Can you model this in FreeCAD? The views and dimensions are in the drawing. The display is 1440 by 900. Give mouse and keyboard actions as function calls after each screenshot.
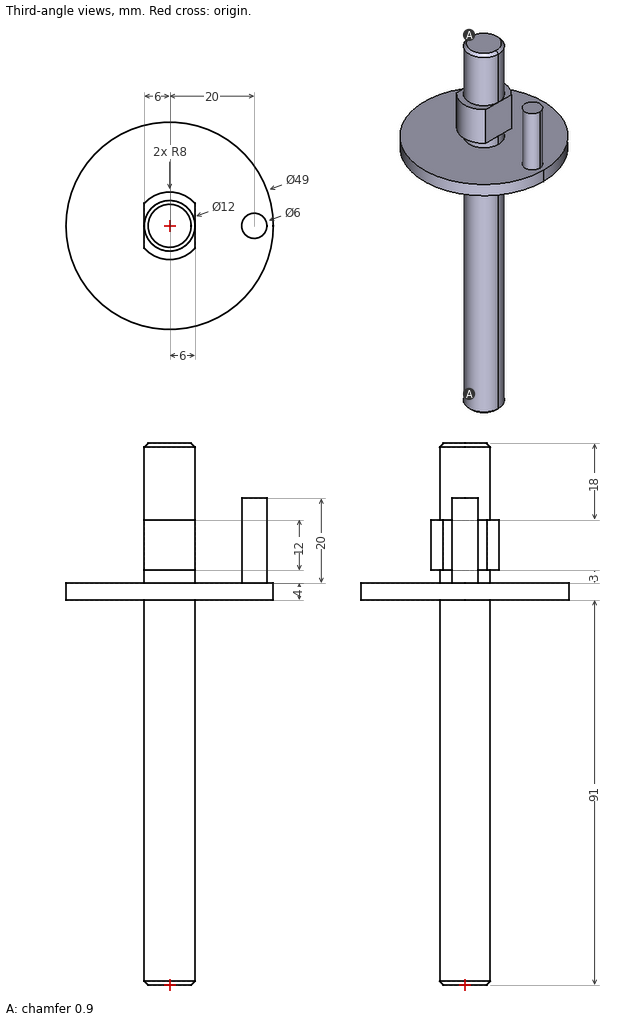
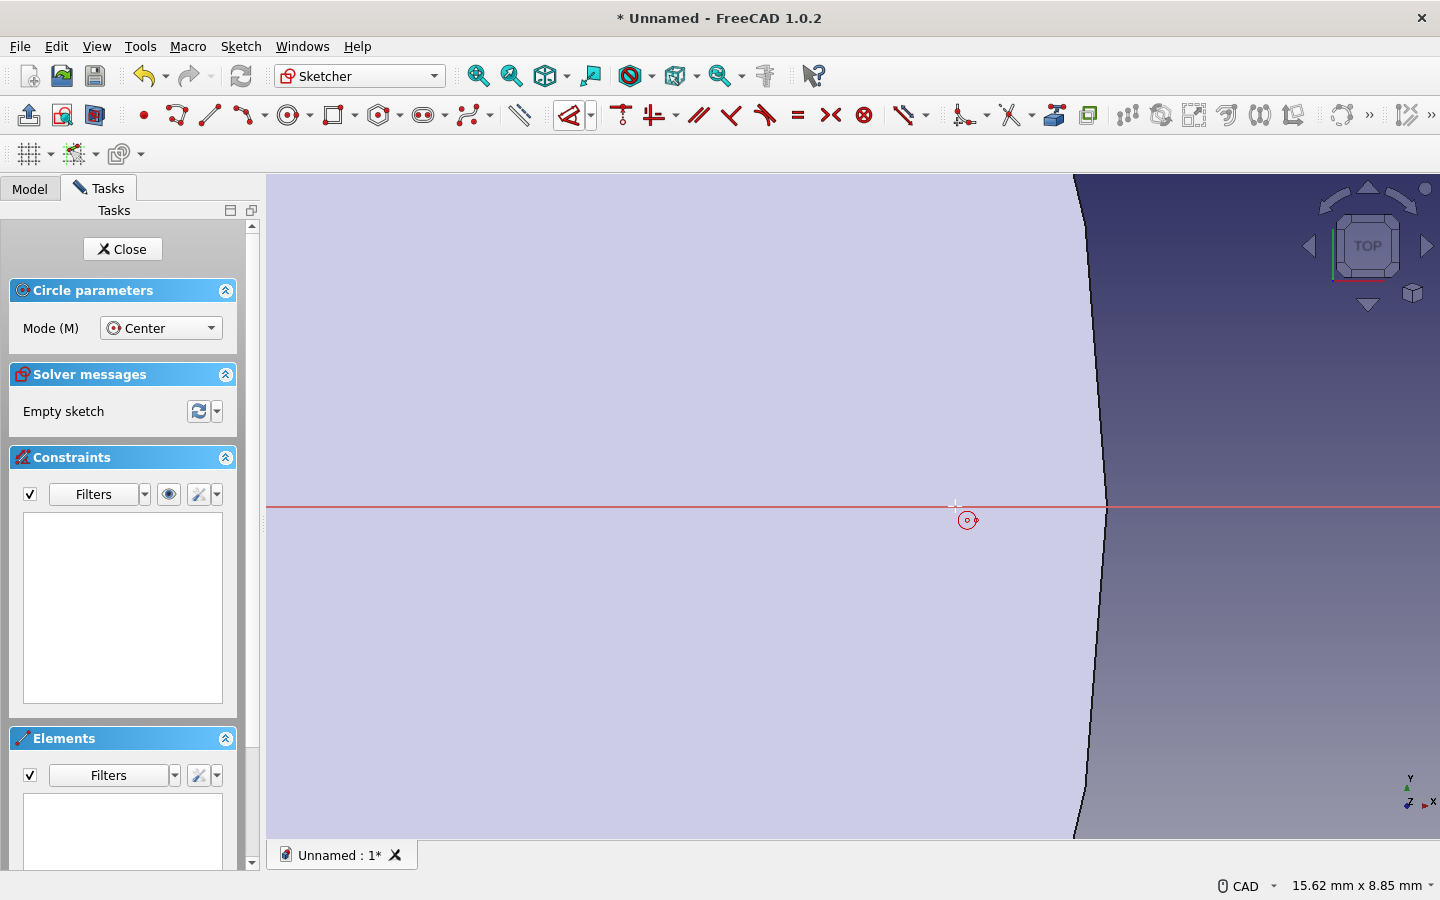
click(769, 506)
click(928, 347)
key(Escape)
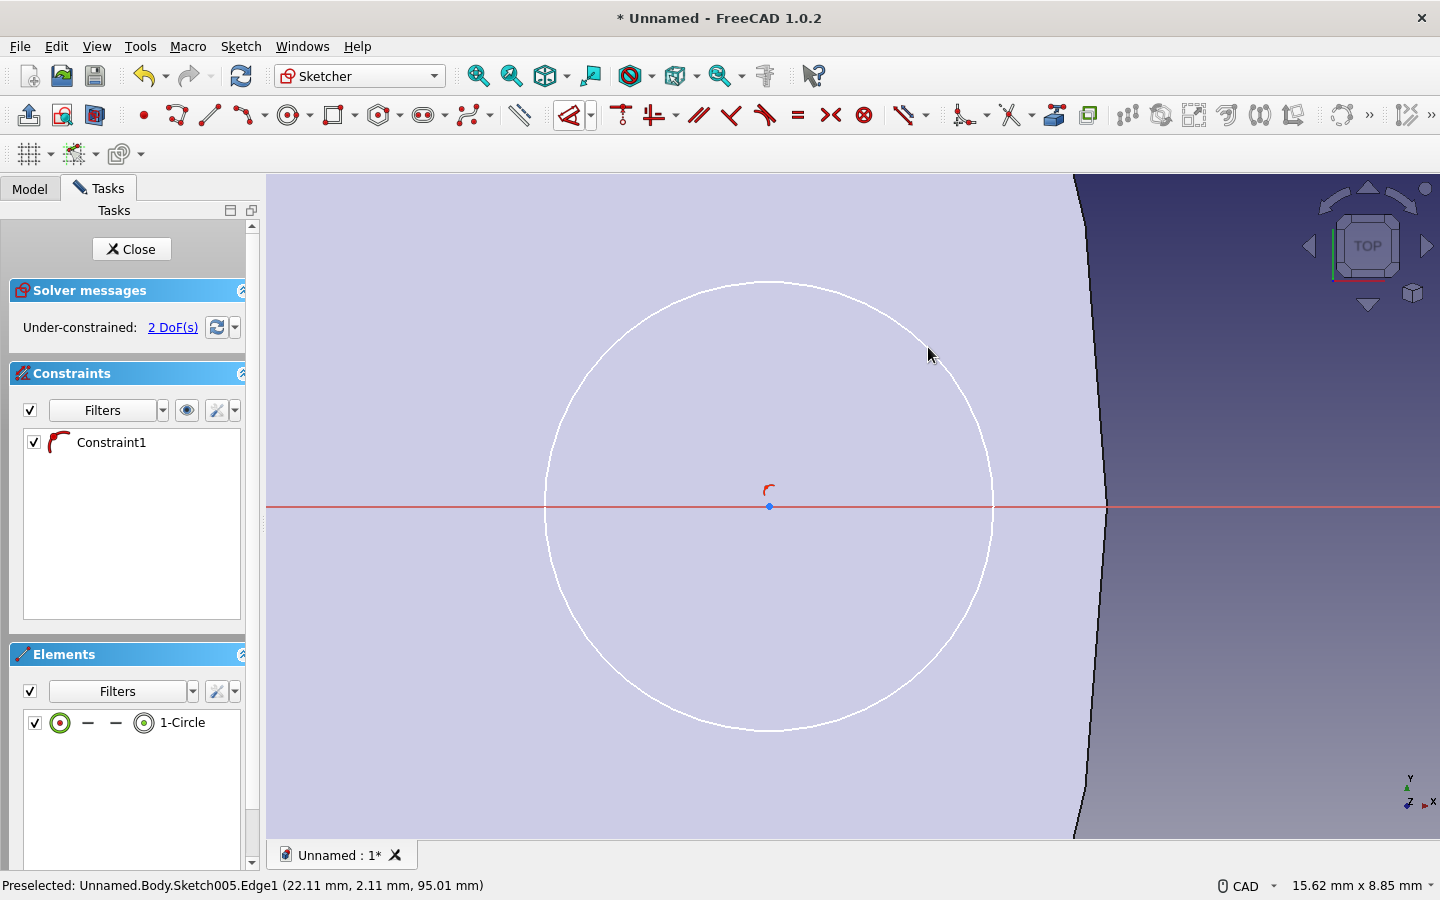
click(927, 347)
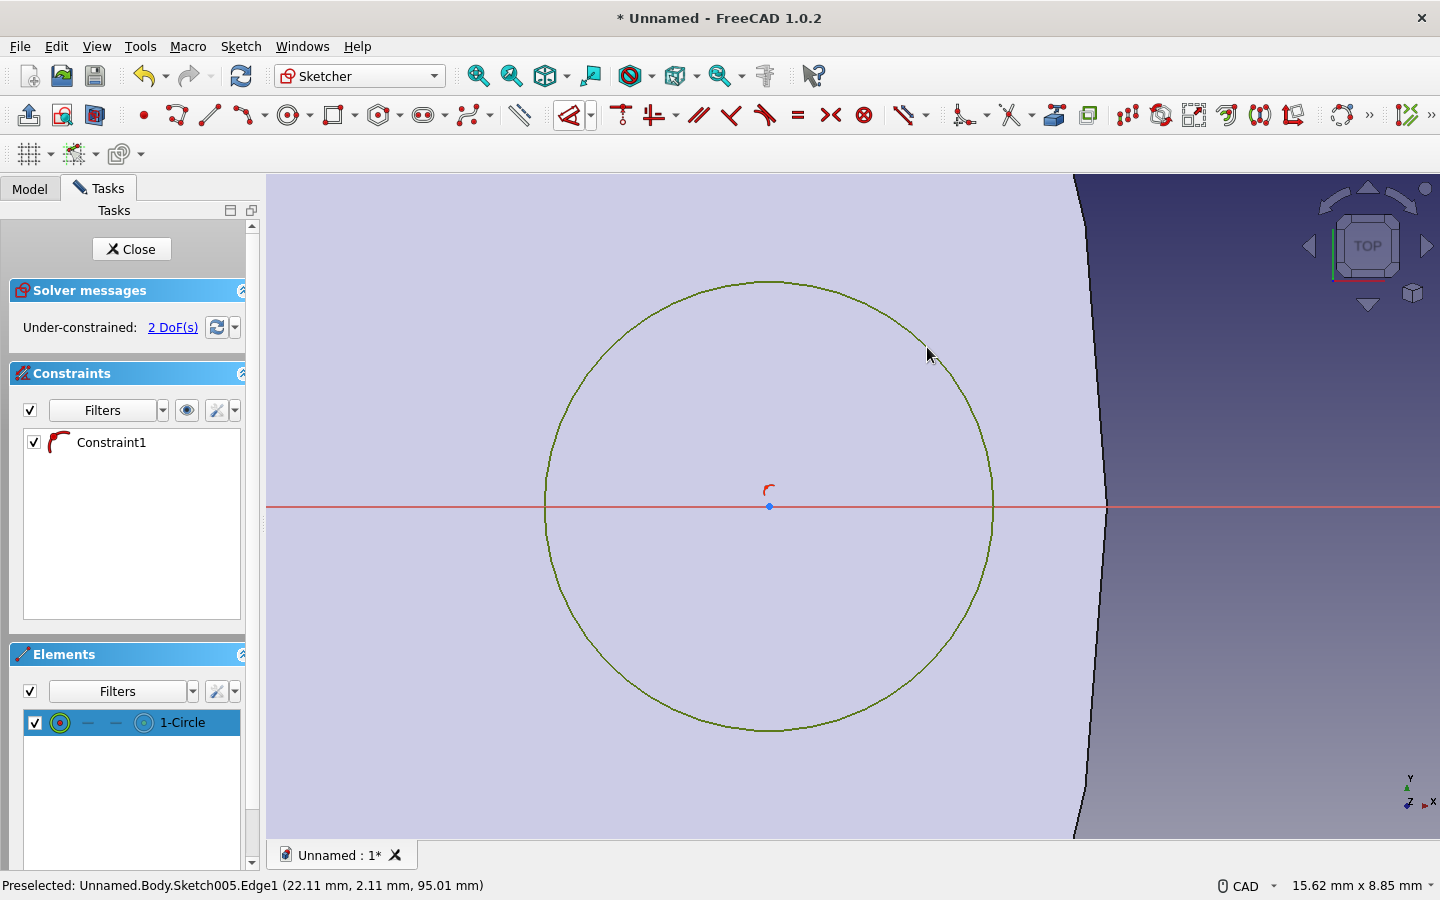
key(k)
key(o)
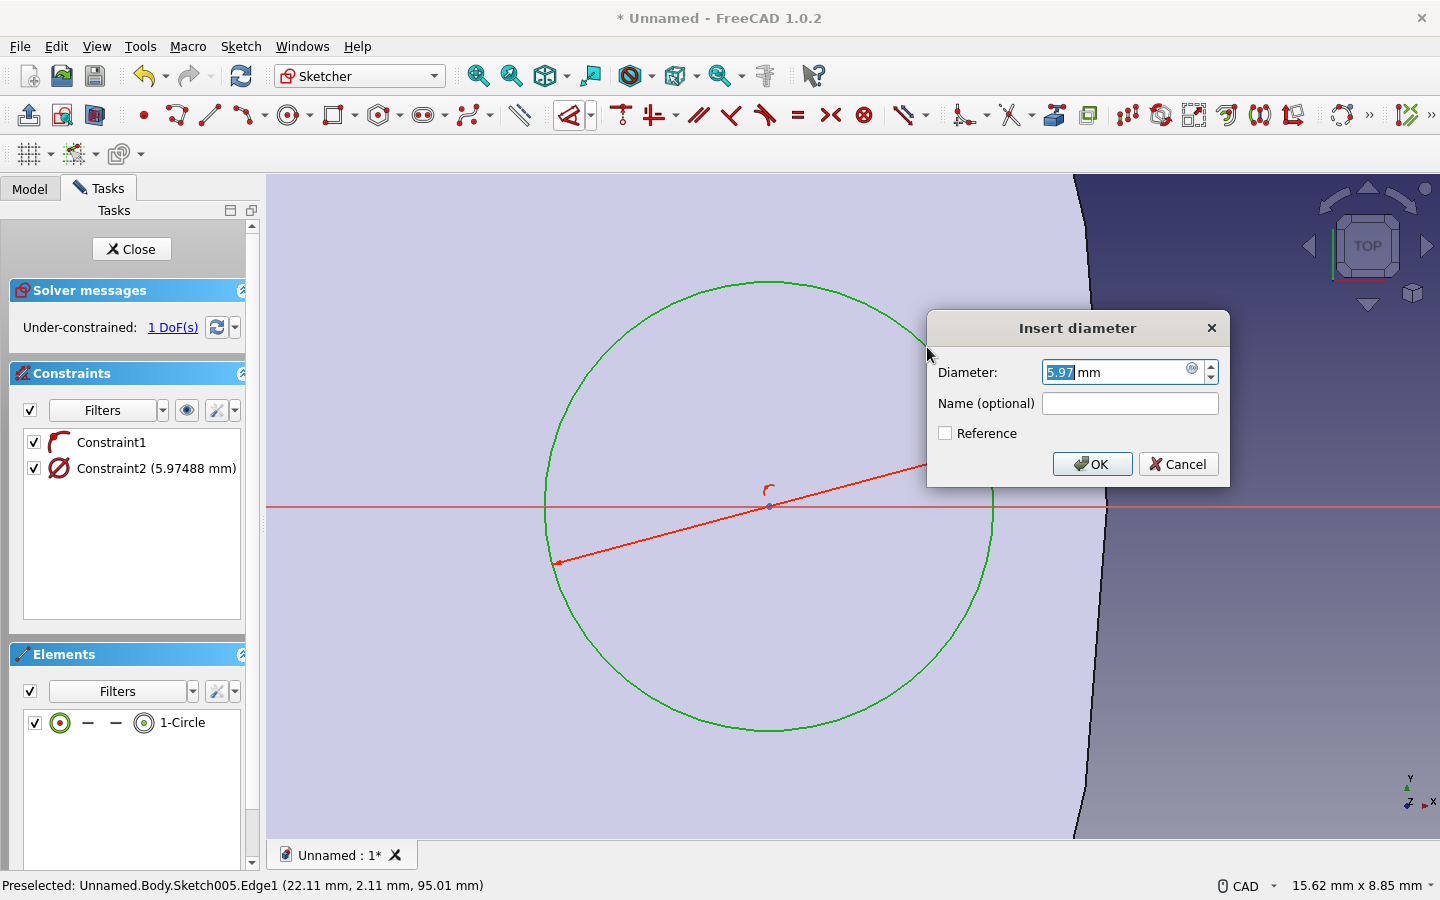
text(6)
key(Return)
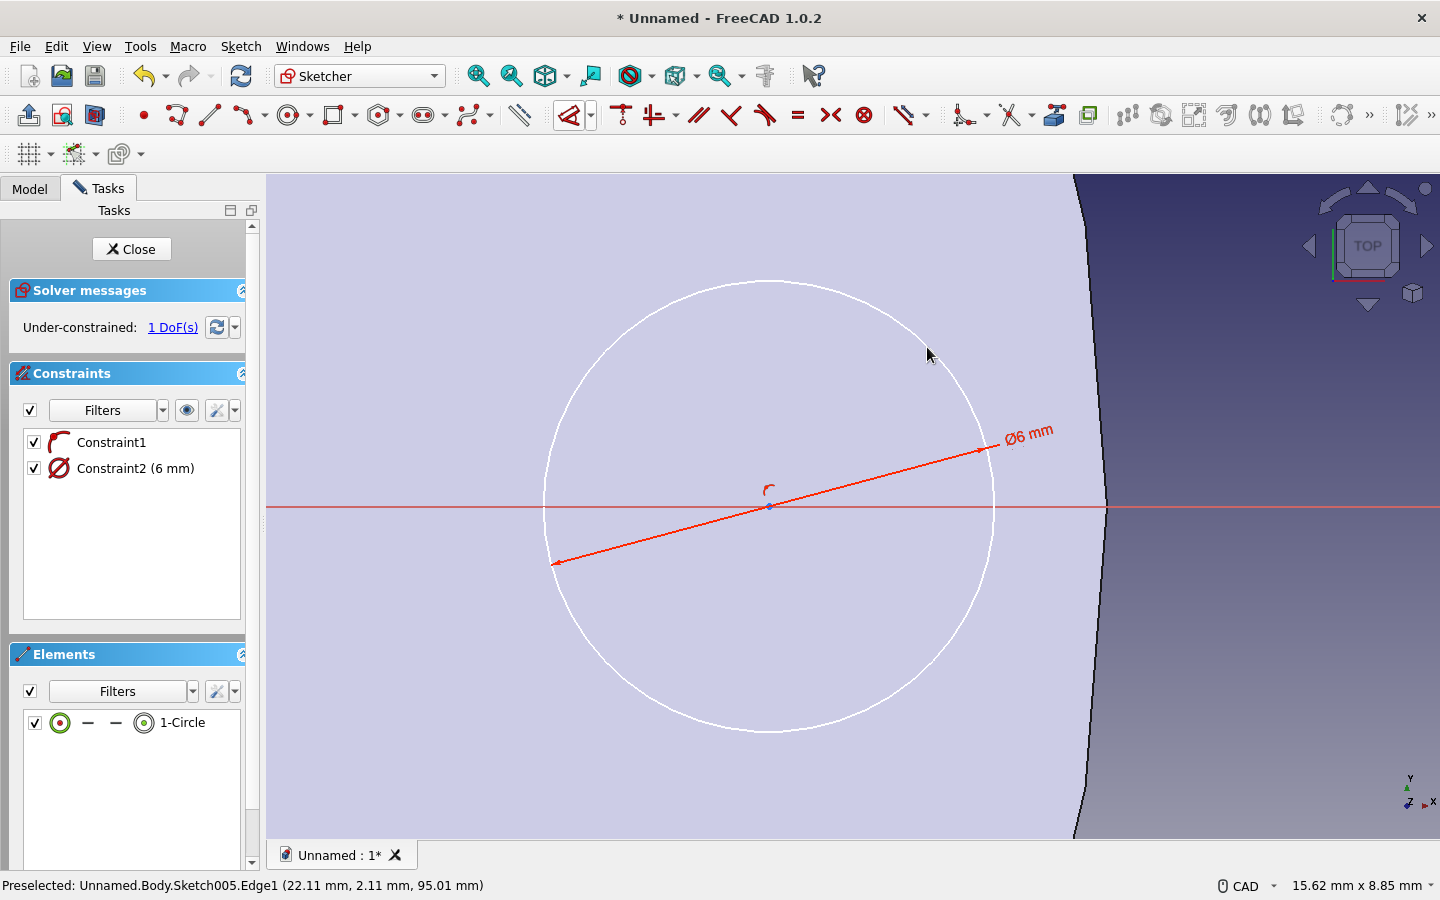
click(769, 506)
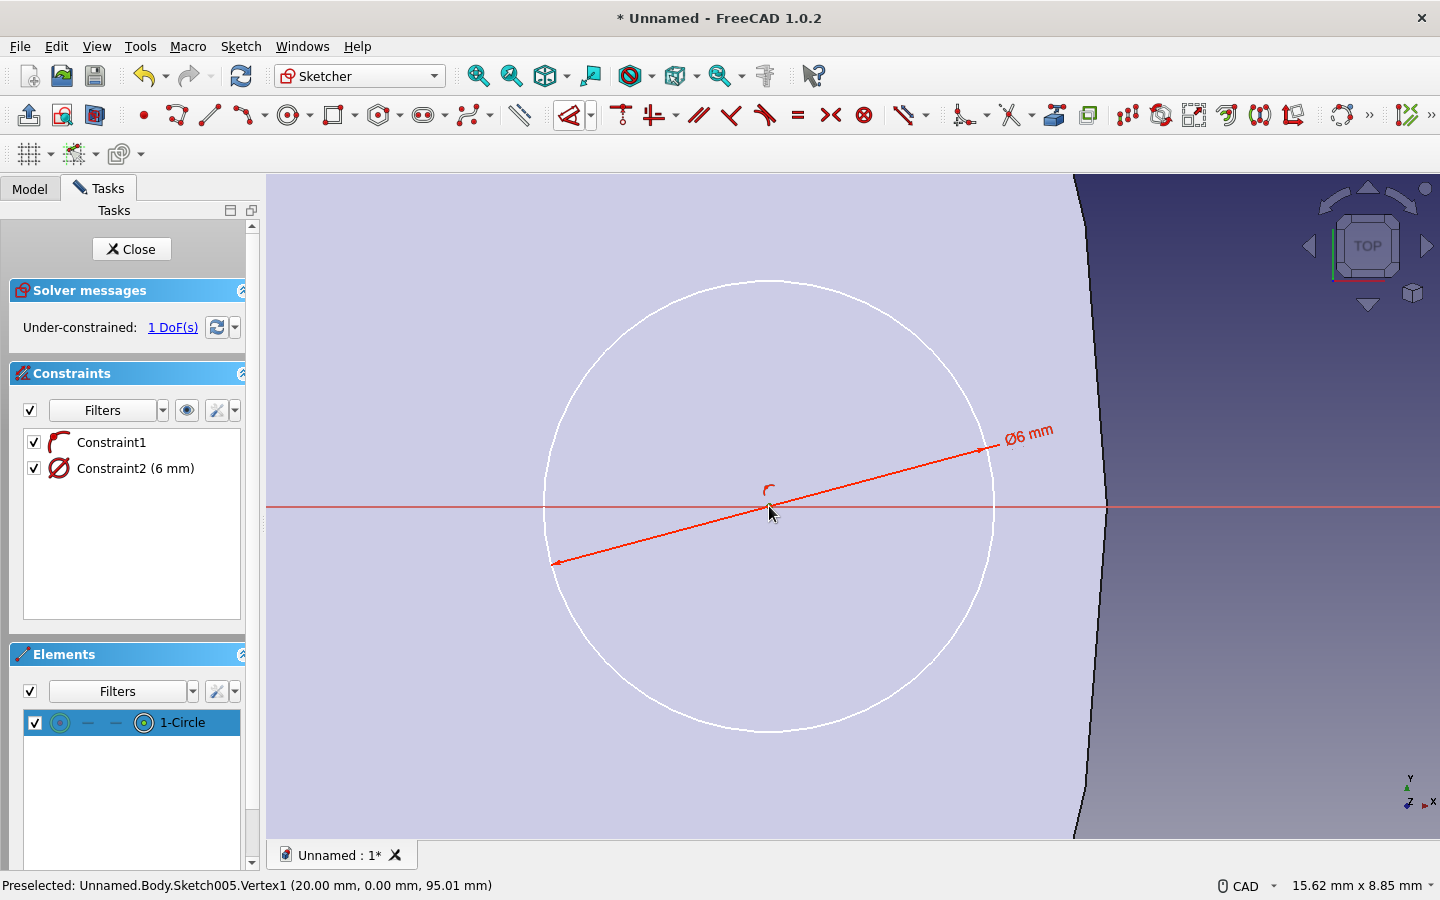
key(l)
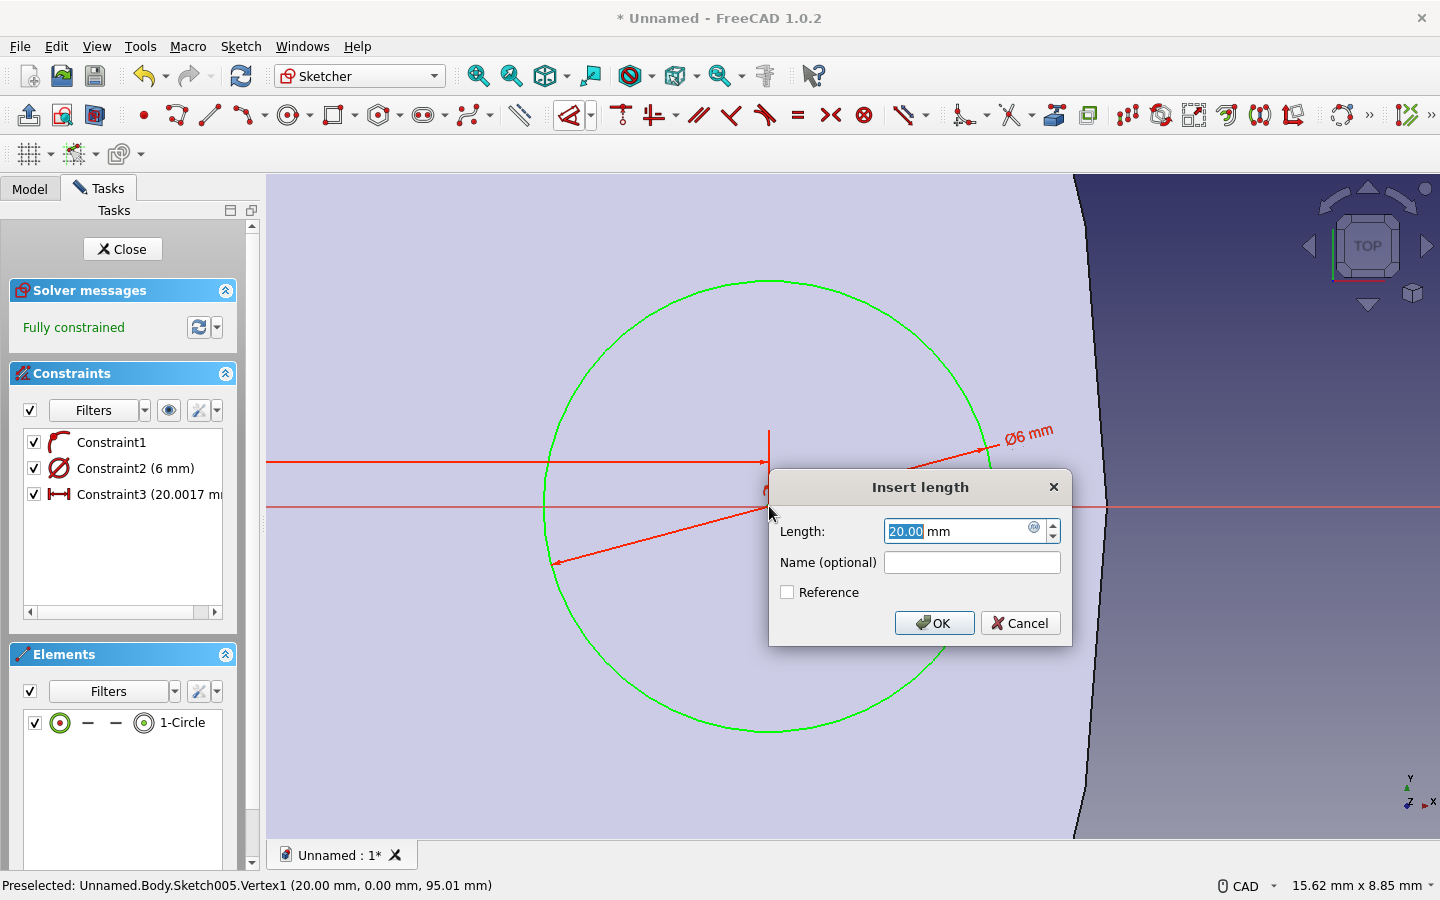
text(20)
key(Return)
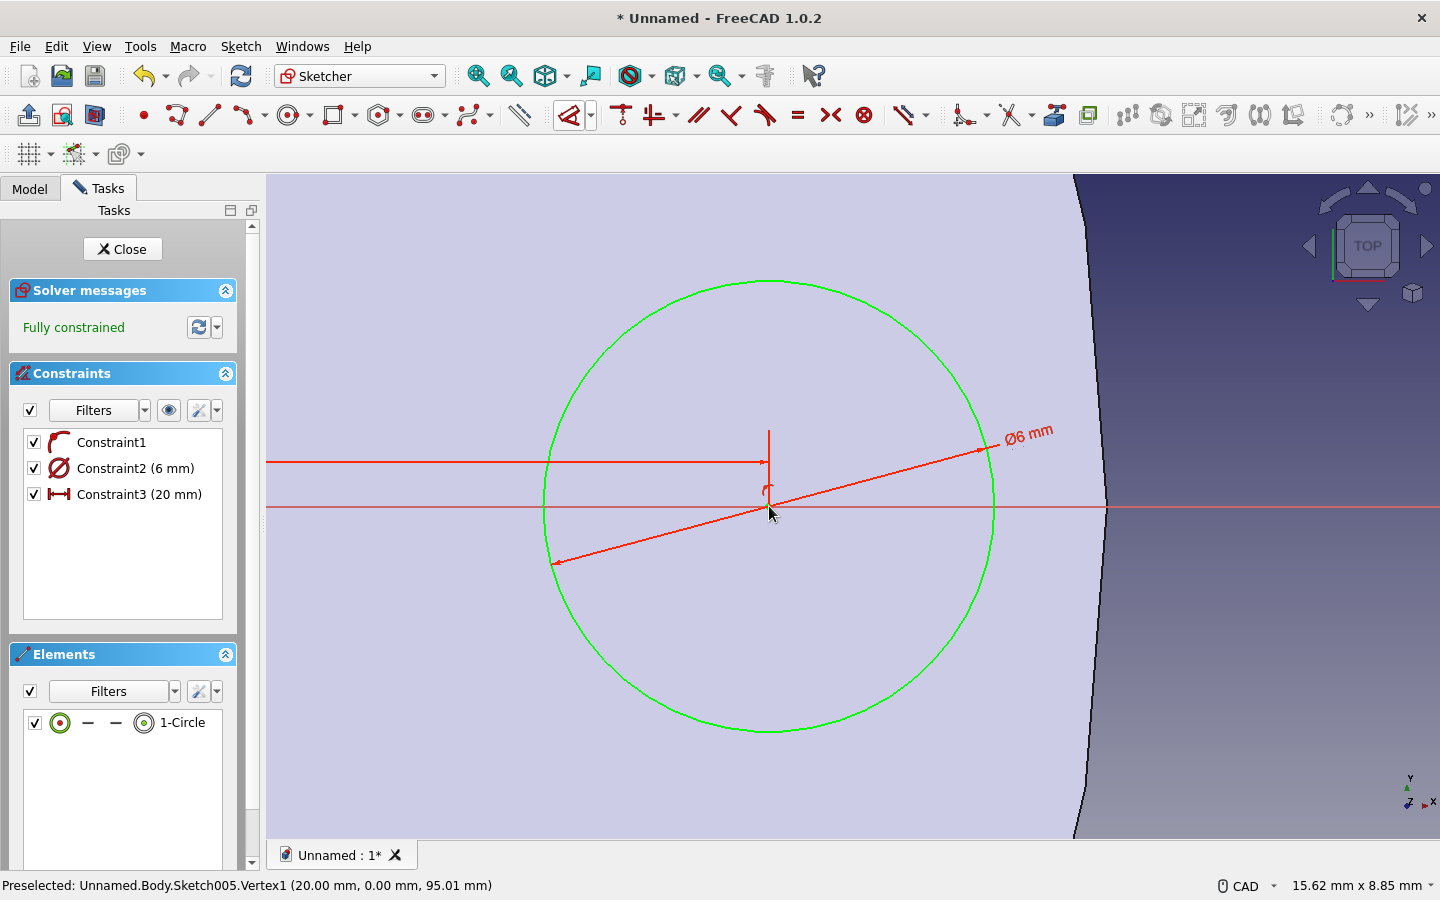
click(123, 249)